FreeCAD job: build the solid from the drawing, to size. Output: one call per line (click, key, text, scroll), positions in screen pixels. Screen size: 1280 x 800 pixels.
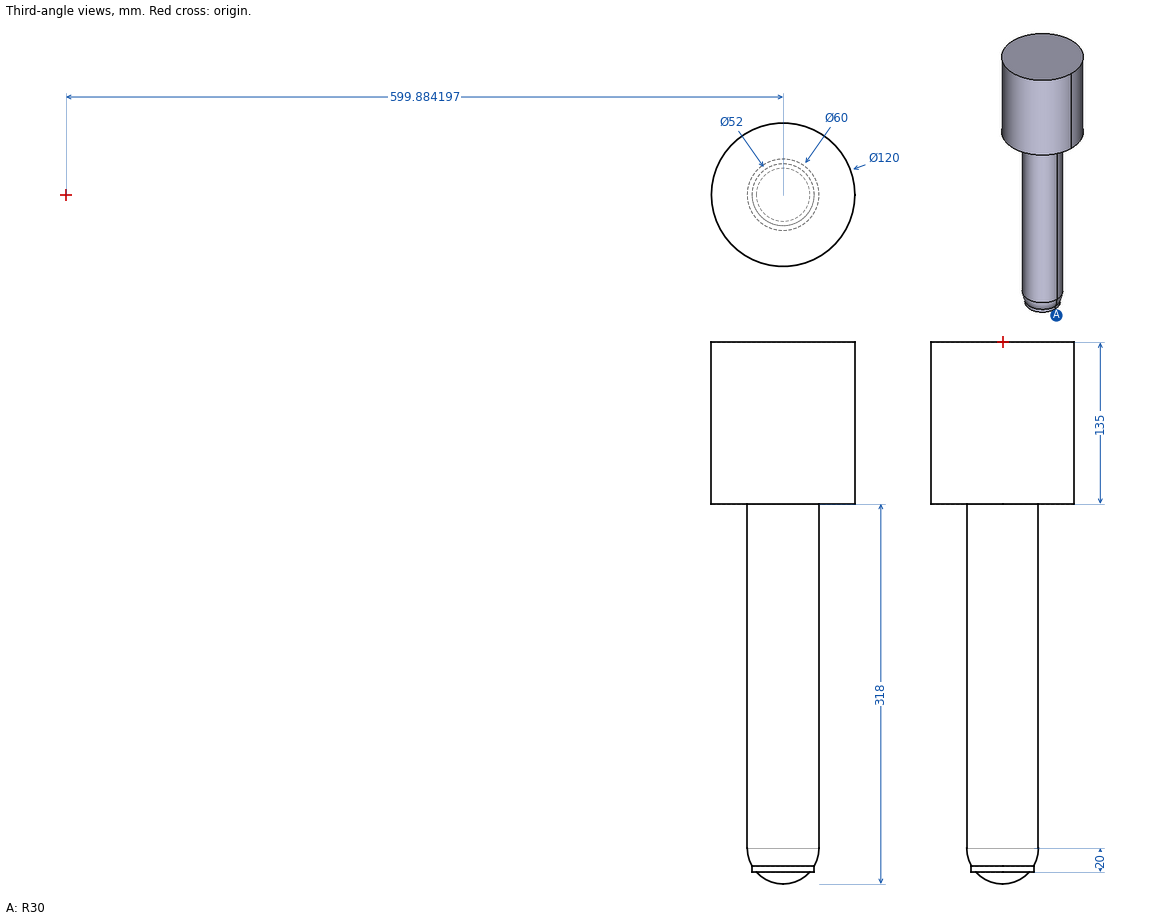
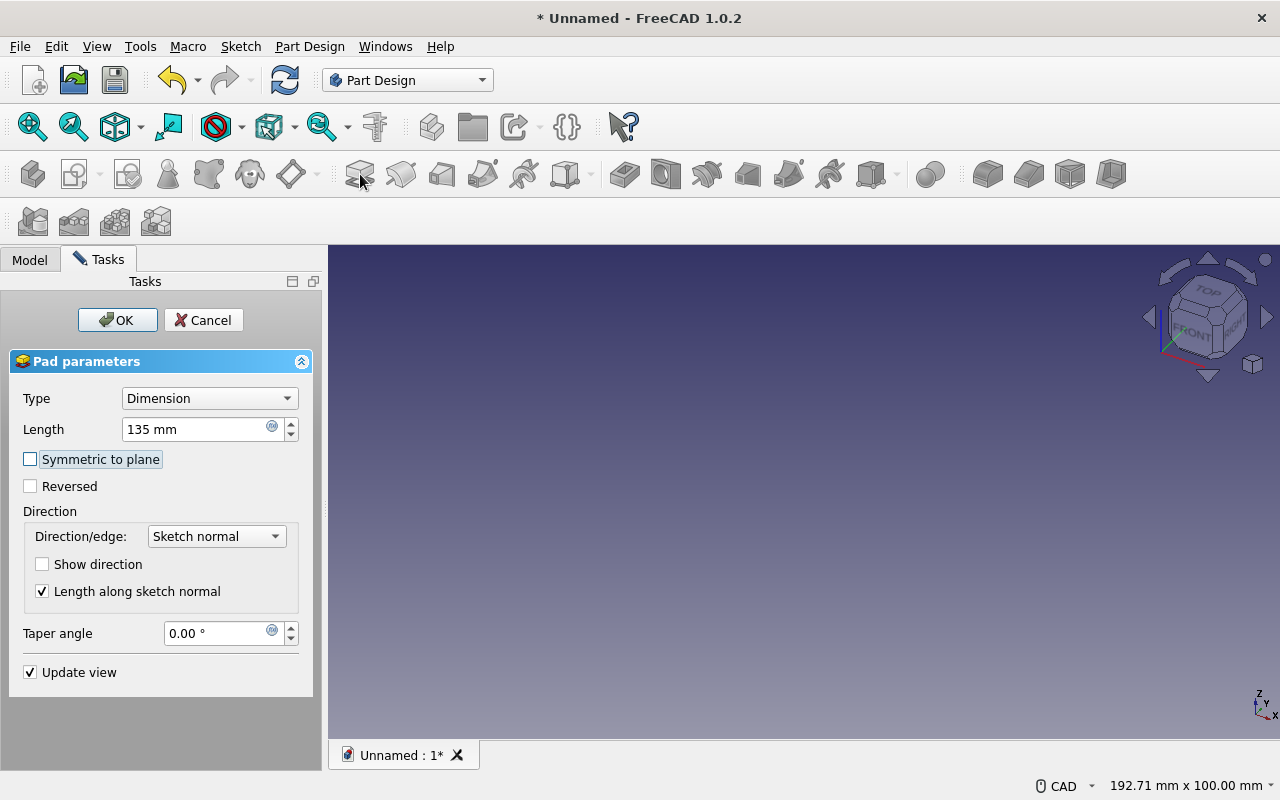
click(31, 486)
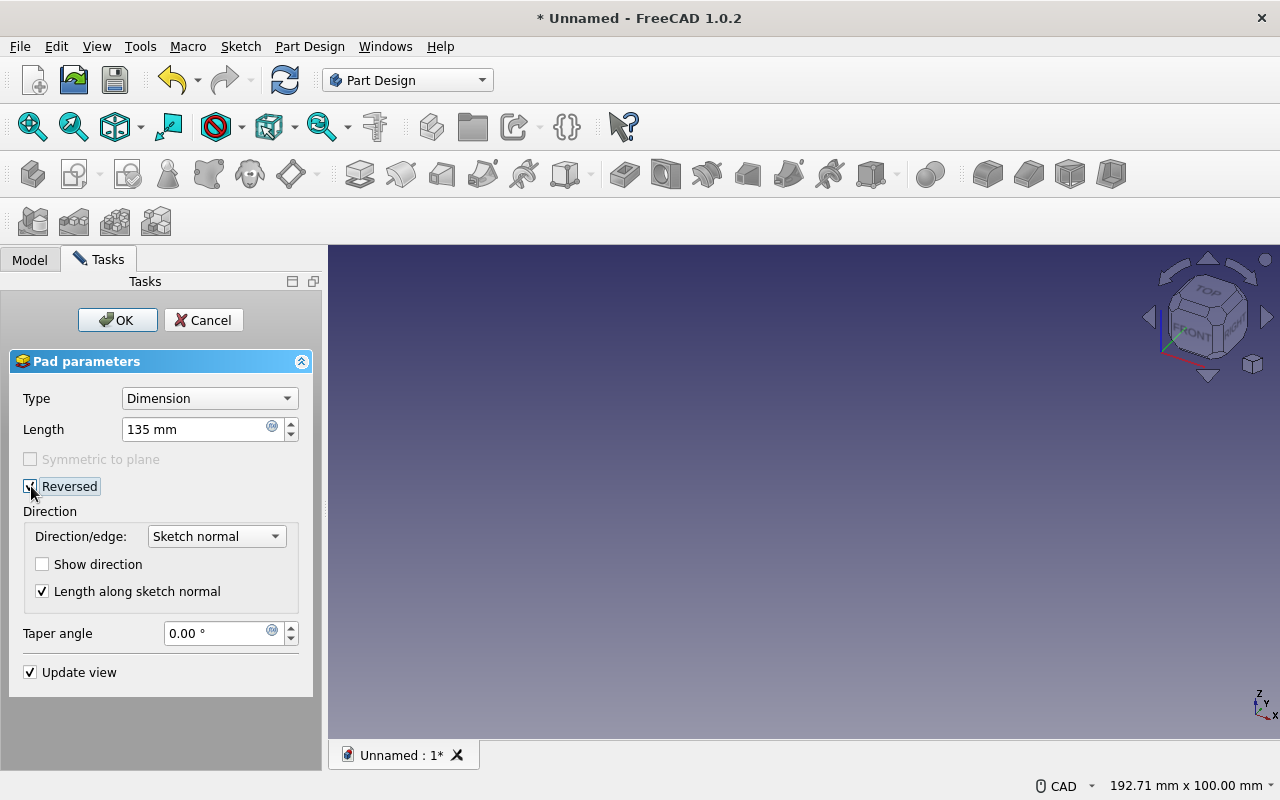
click(118, 320)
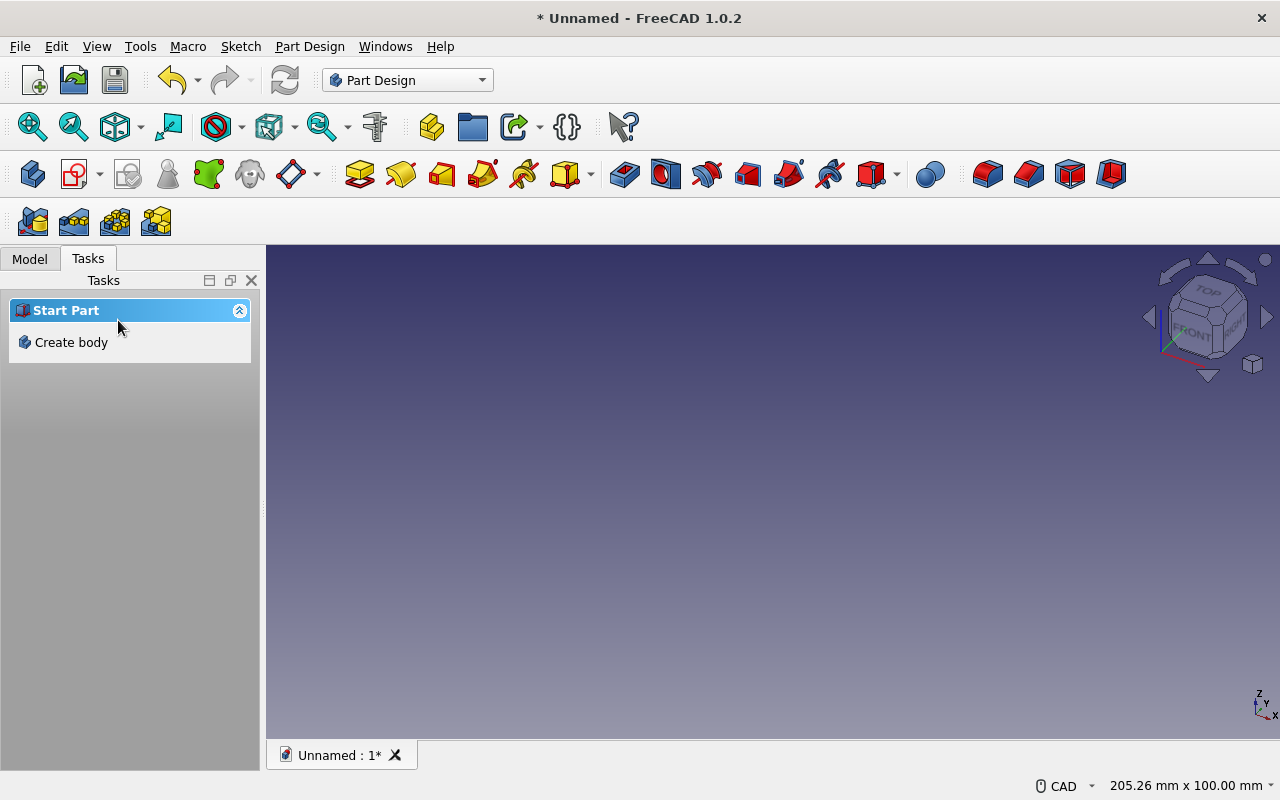
key(v)
key(f)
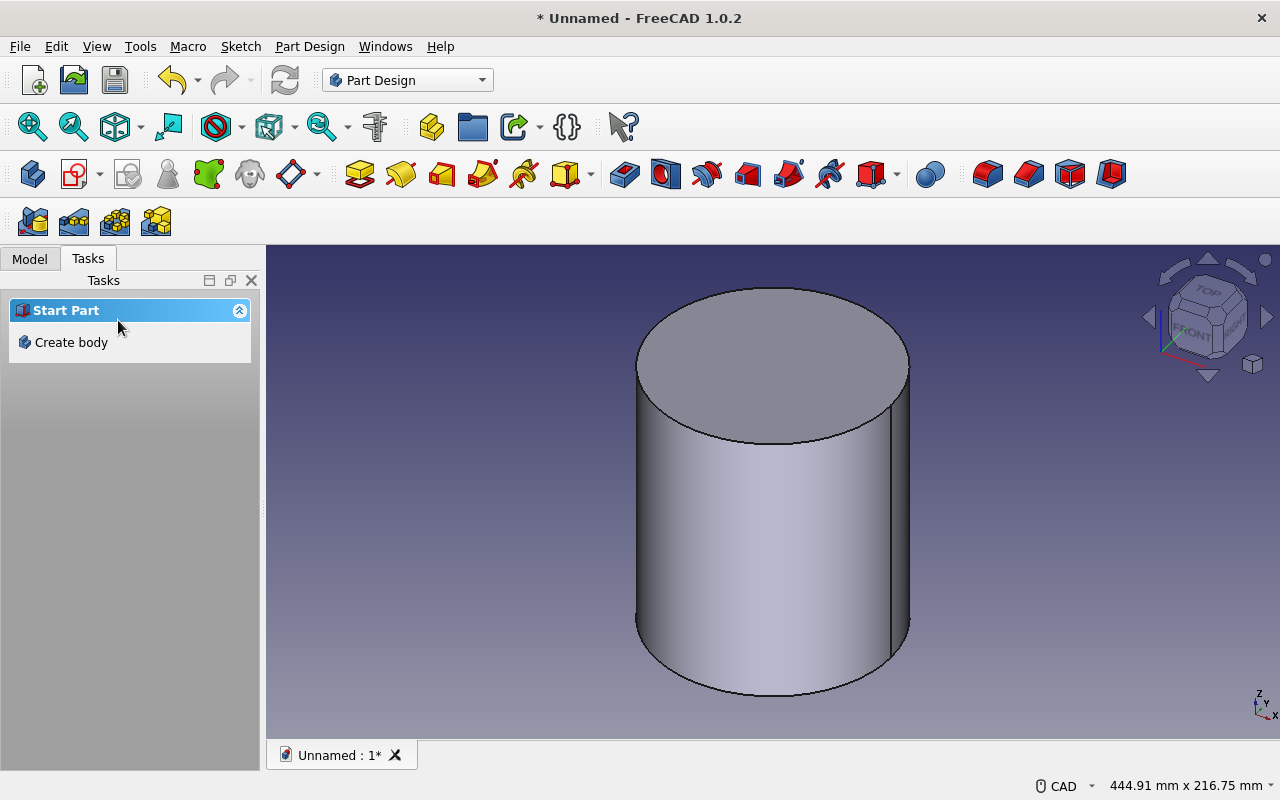
key(5)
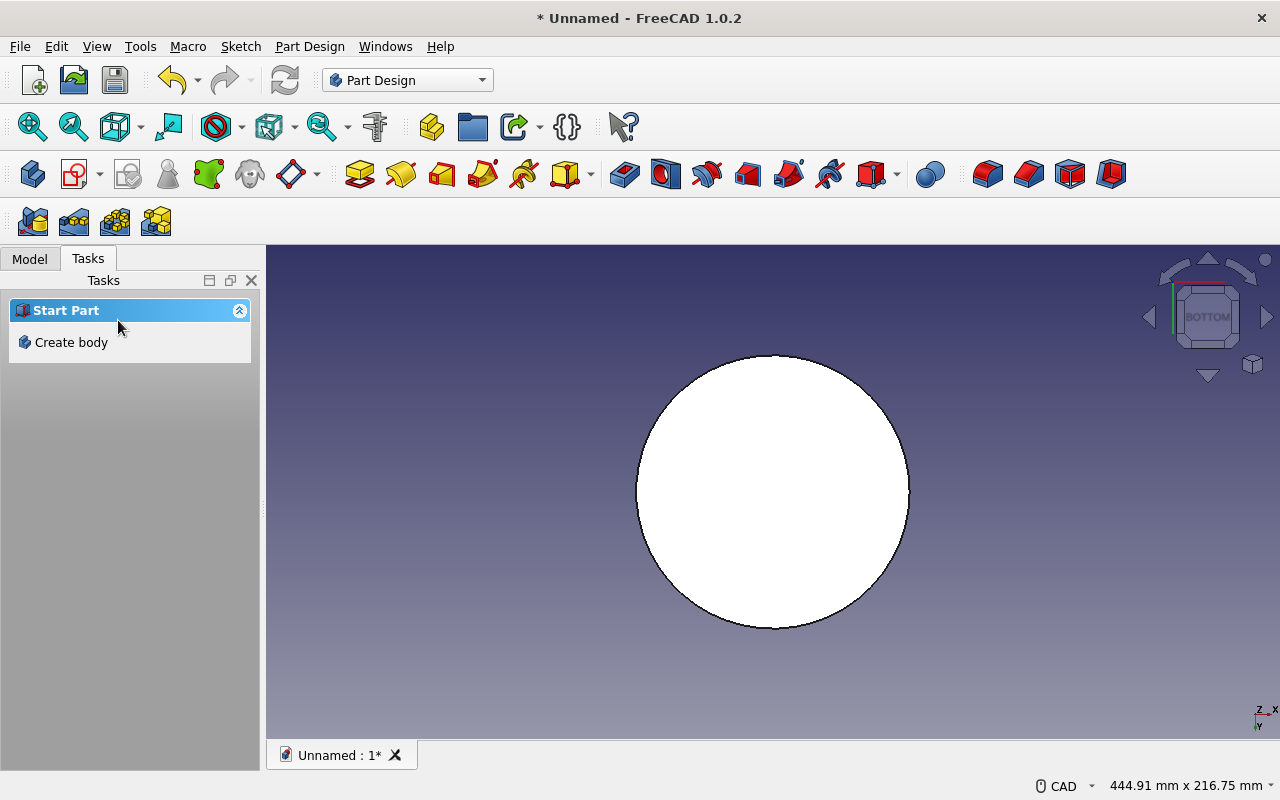
click(773, 491)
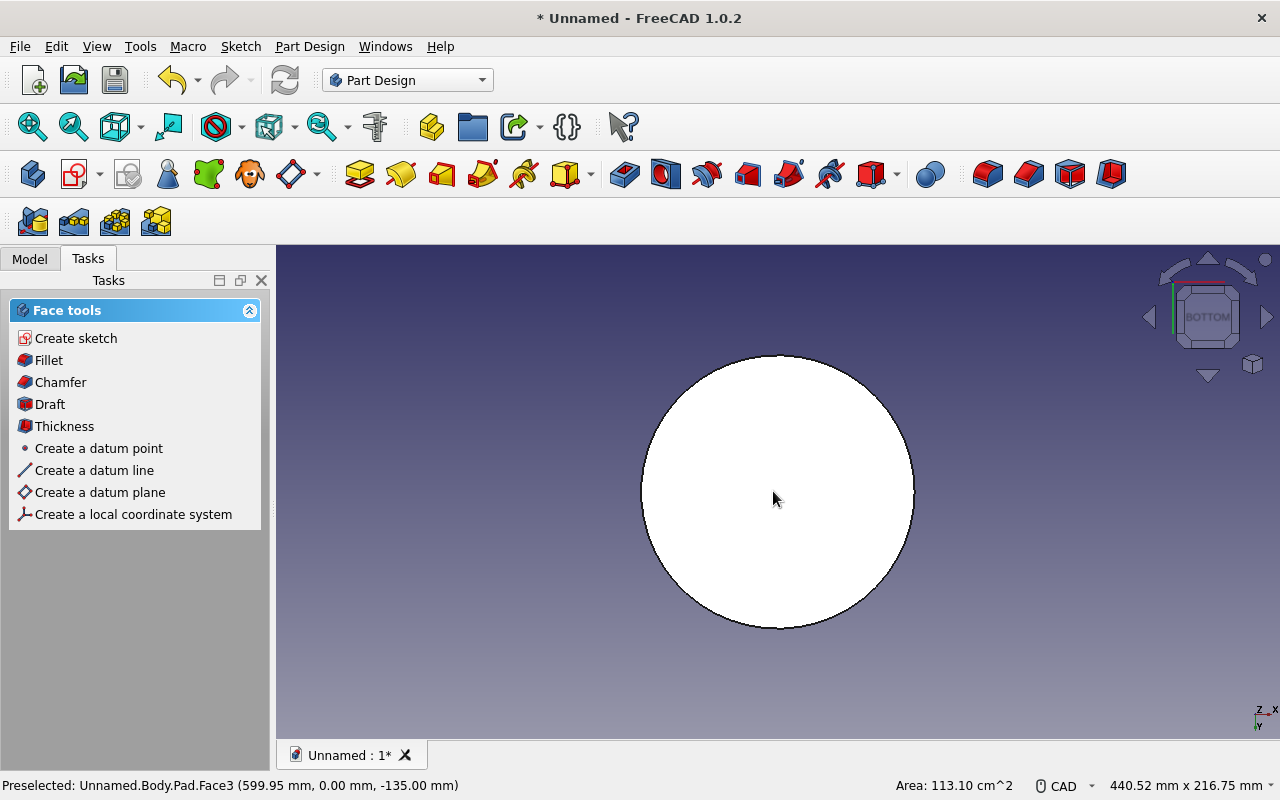
click(74, 174)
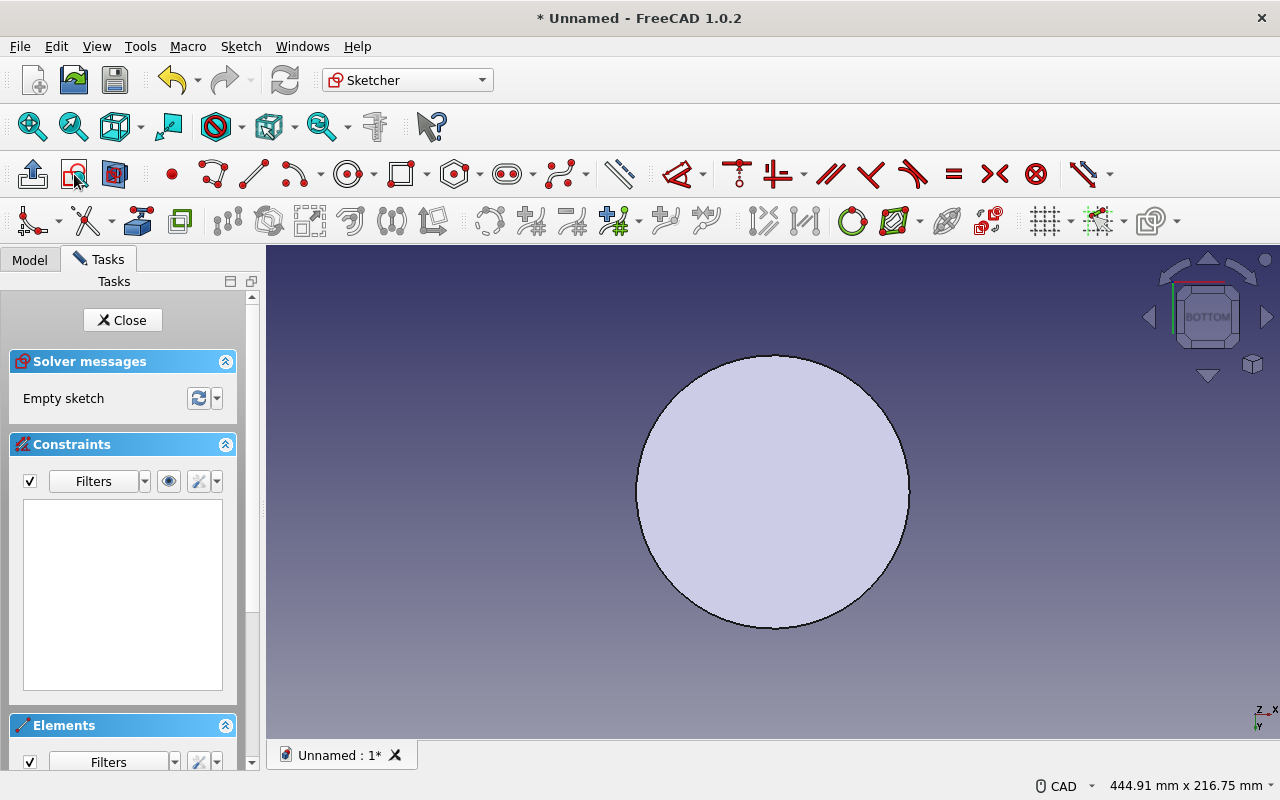
scroll(829, 492, up, 4)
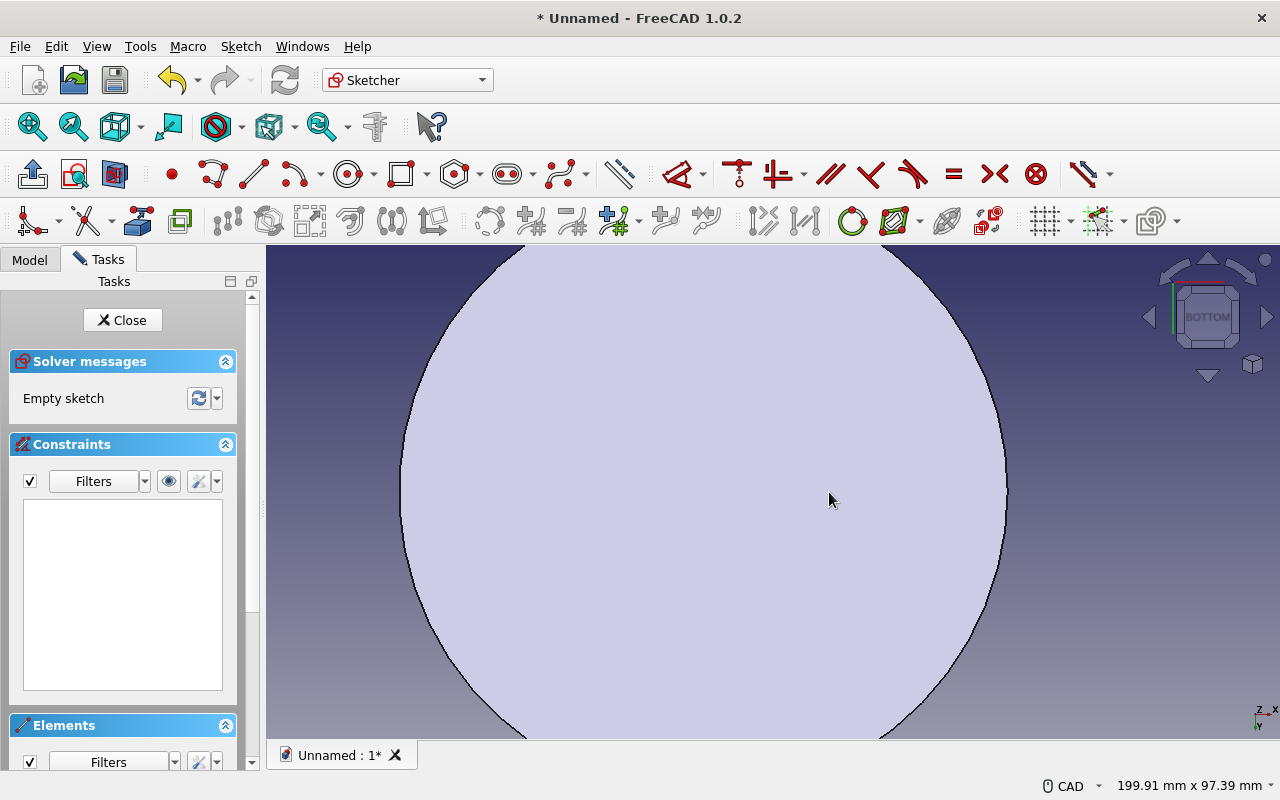
click(348, 174)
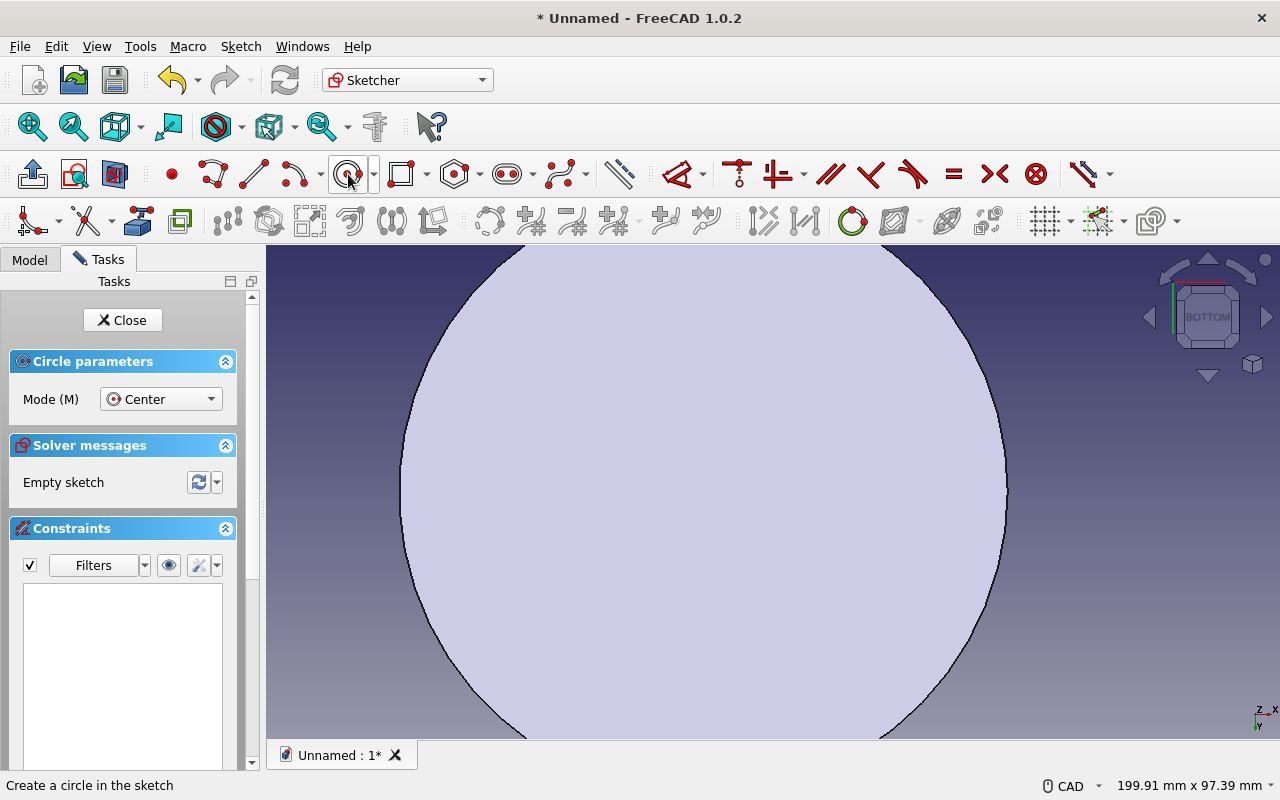
click(703, 491)
move(811, 384)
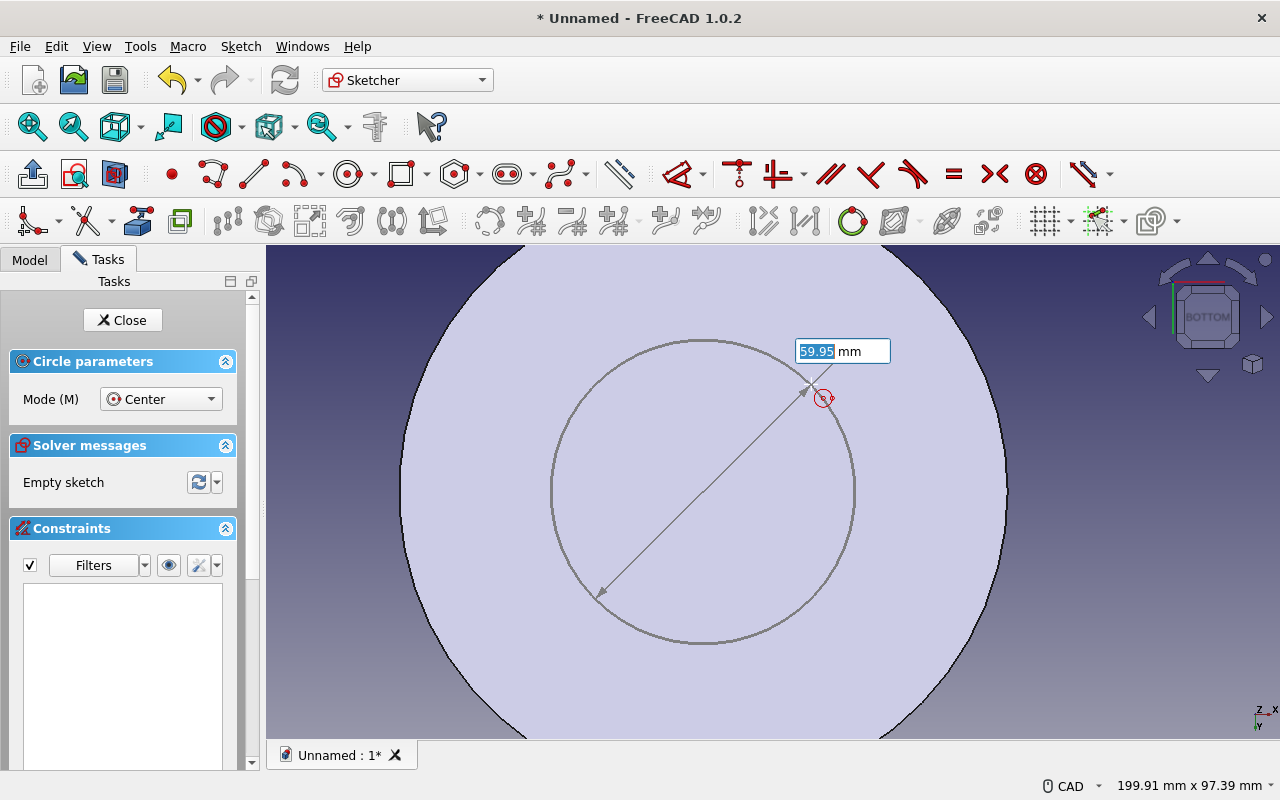
text(60)
key(Return)
key(Escape)